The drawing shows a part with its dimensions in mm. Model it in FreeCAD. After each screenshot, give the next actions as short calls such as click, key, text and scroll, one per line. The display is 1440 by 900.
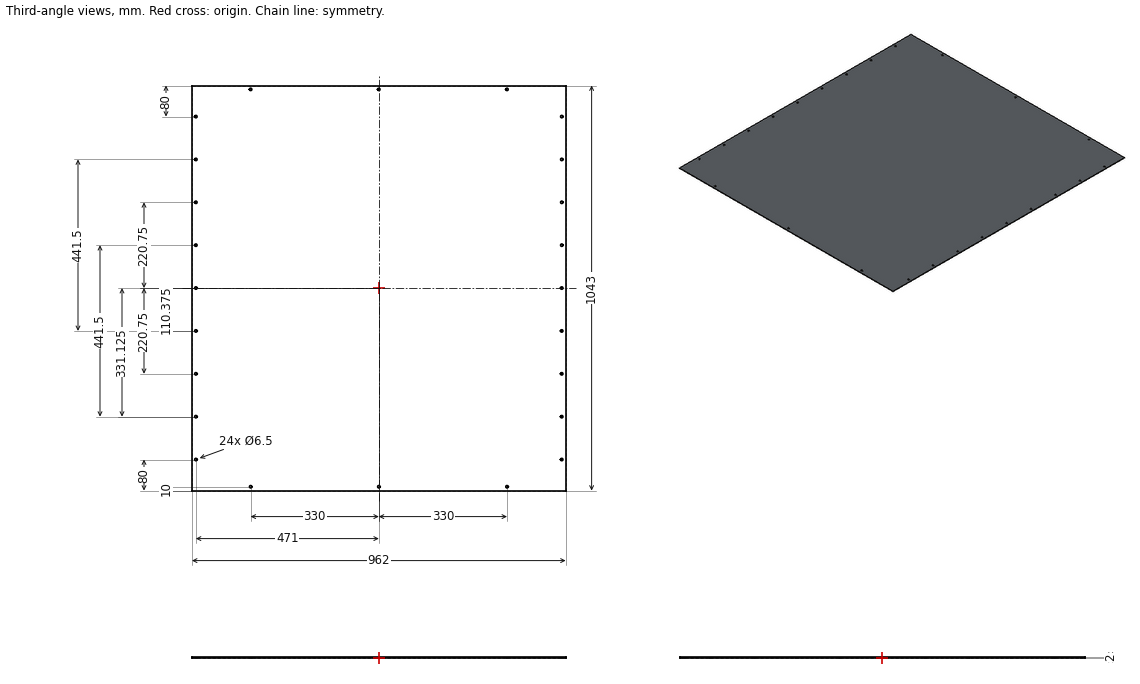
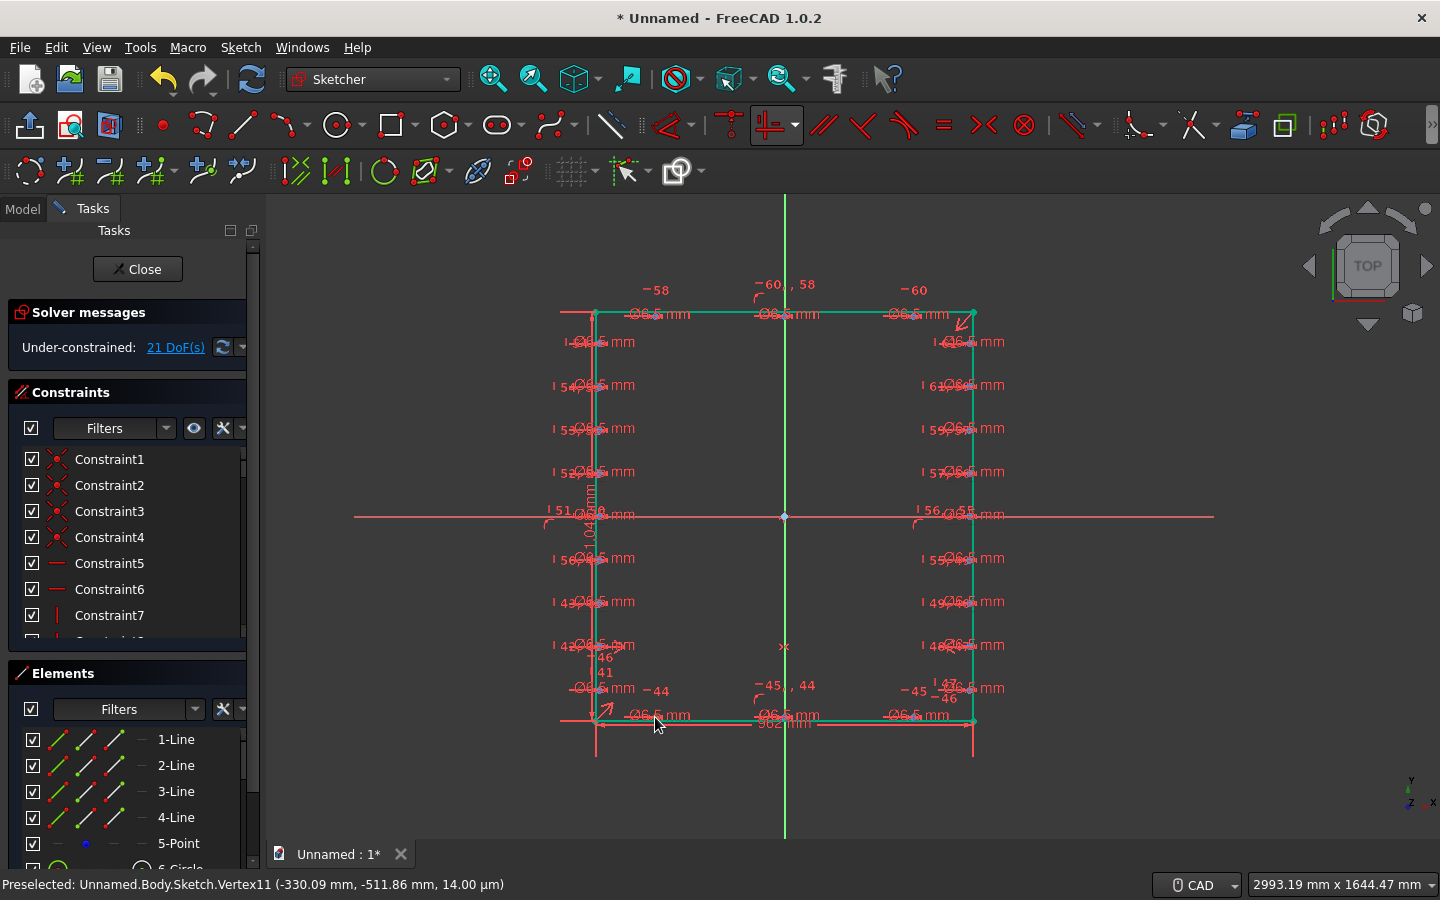
click(655, 316)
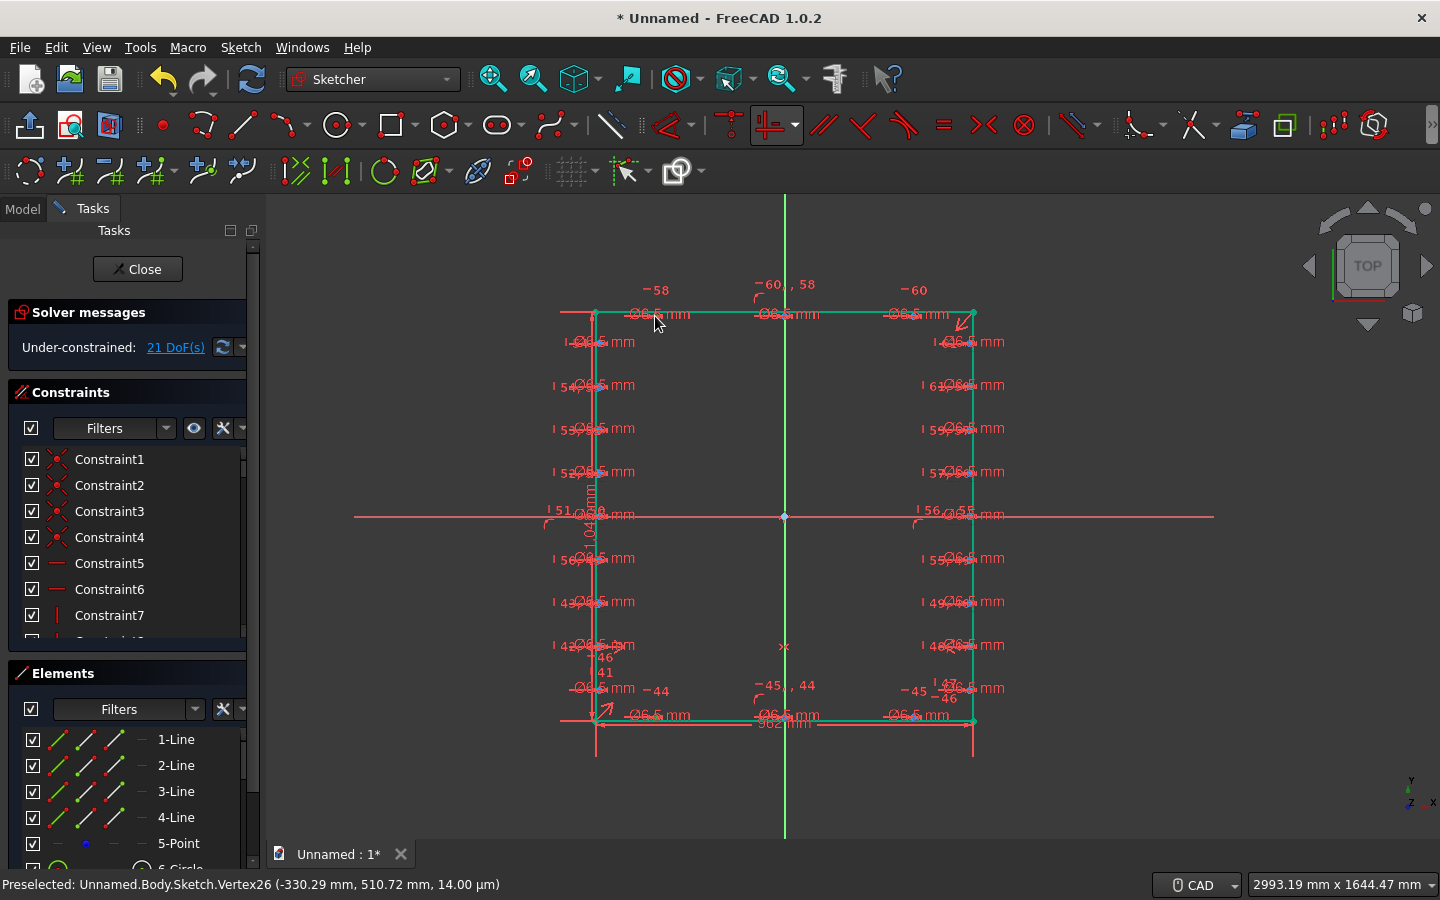
click(364, 517)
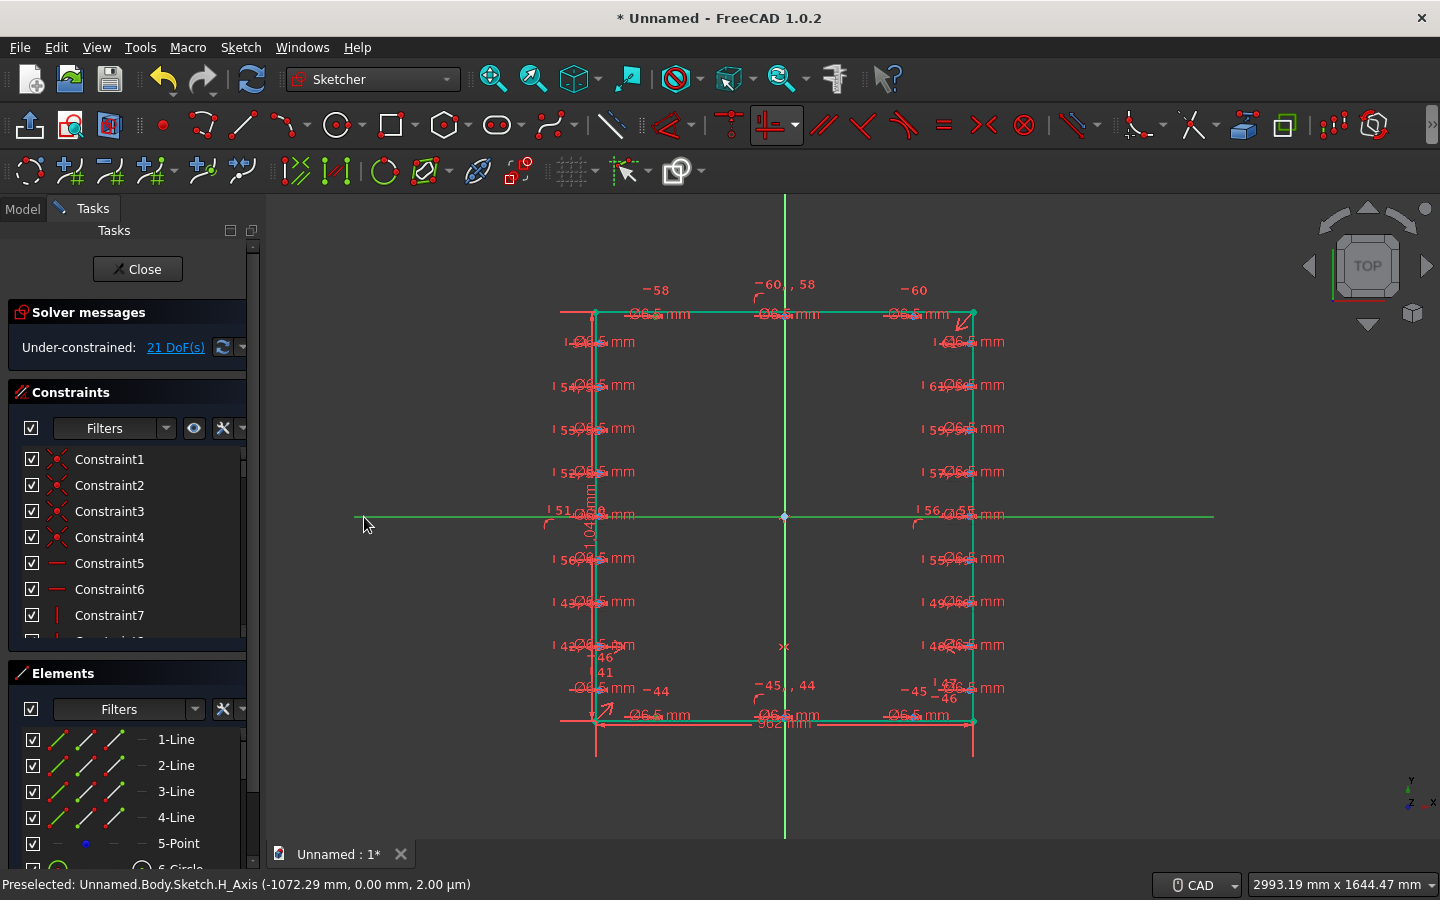
click(984, 126)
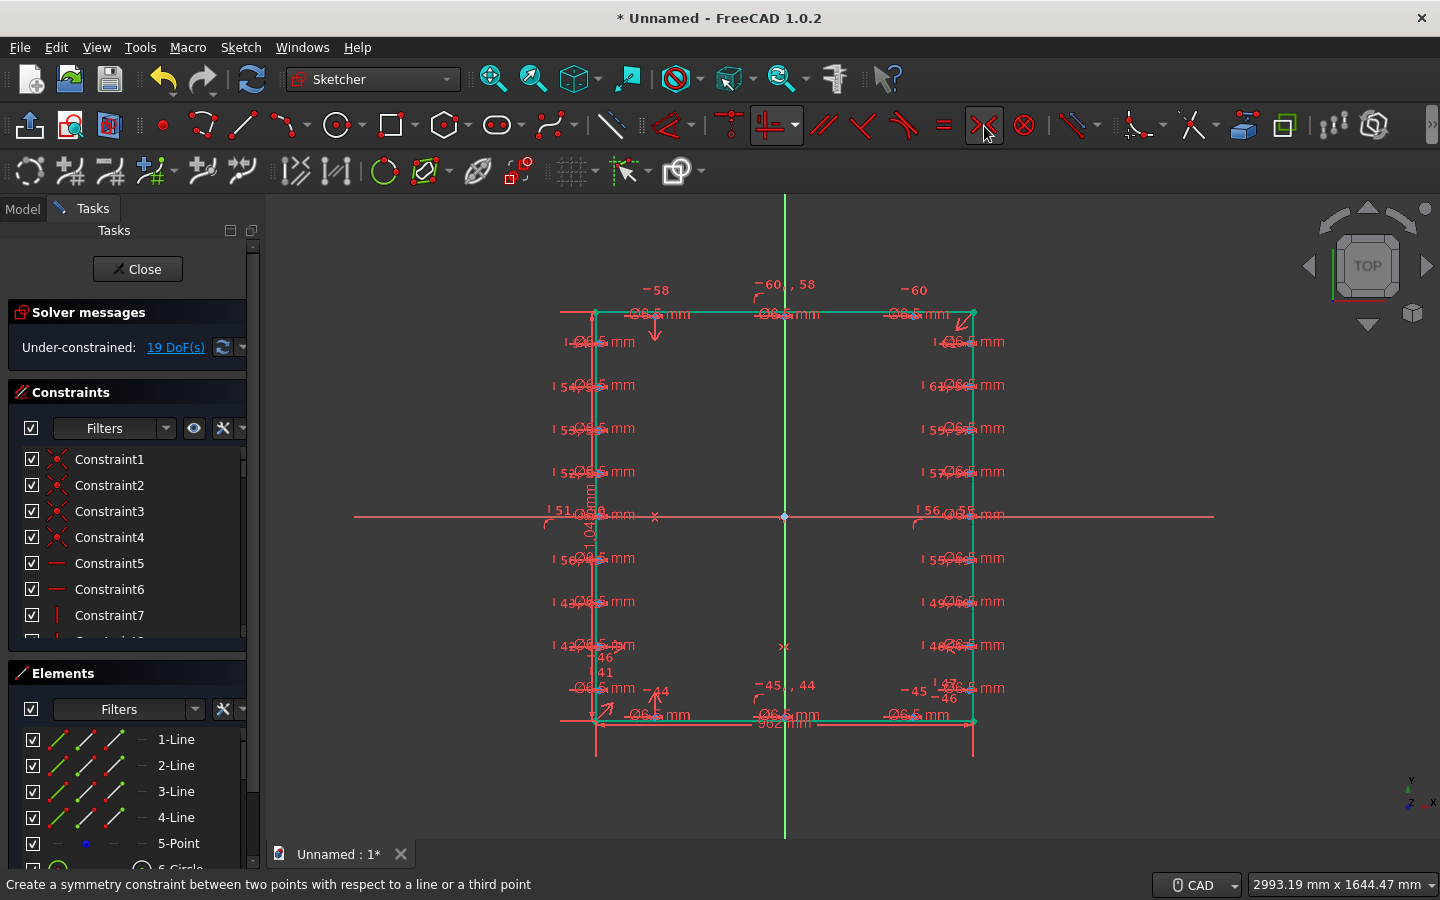
click(666, 126)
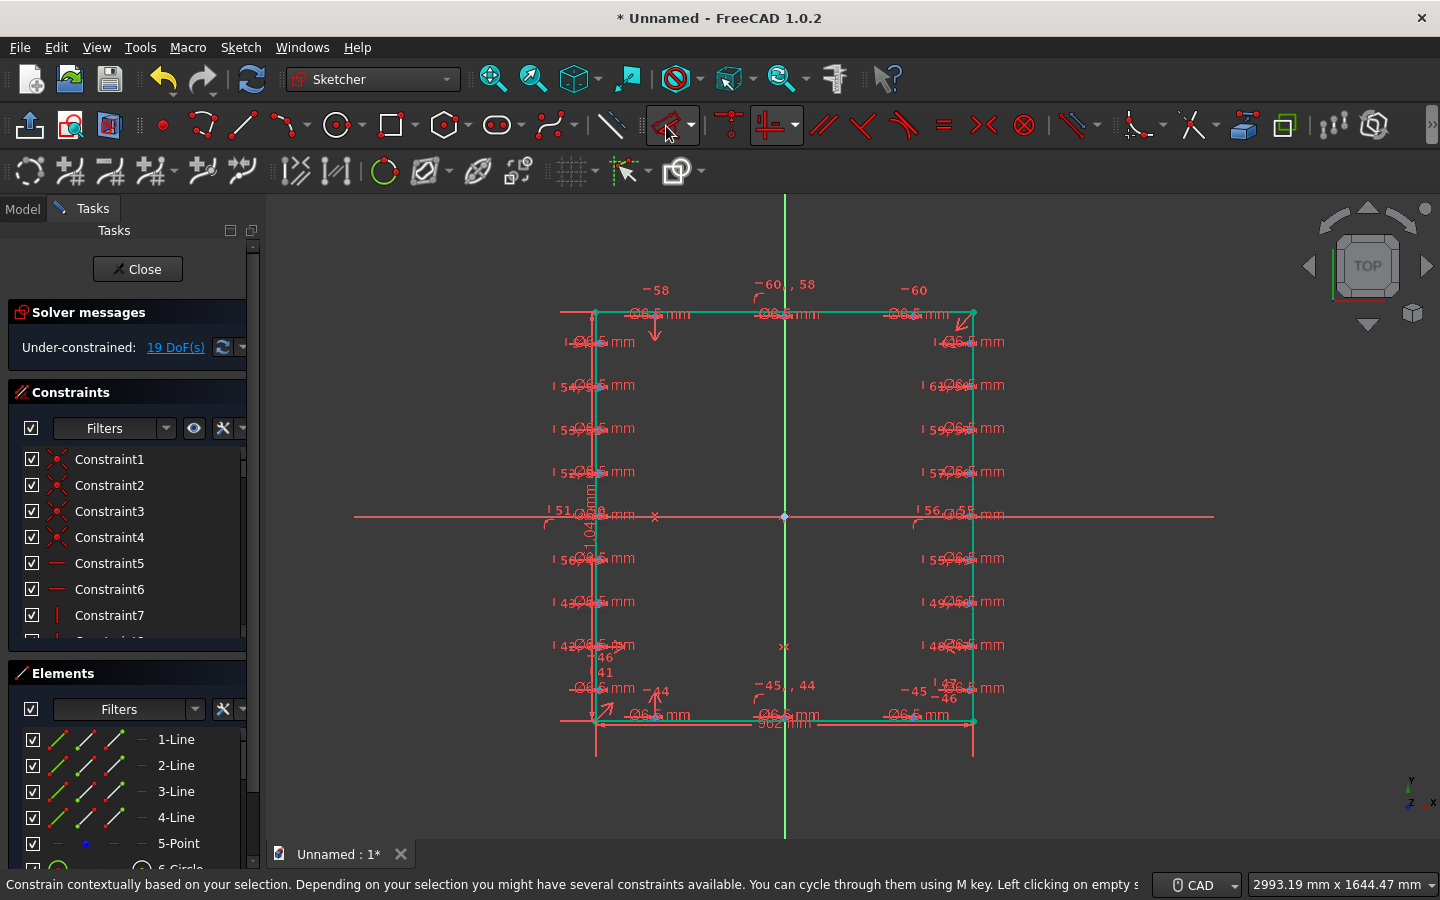
click(600, 690)
click(692, 483)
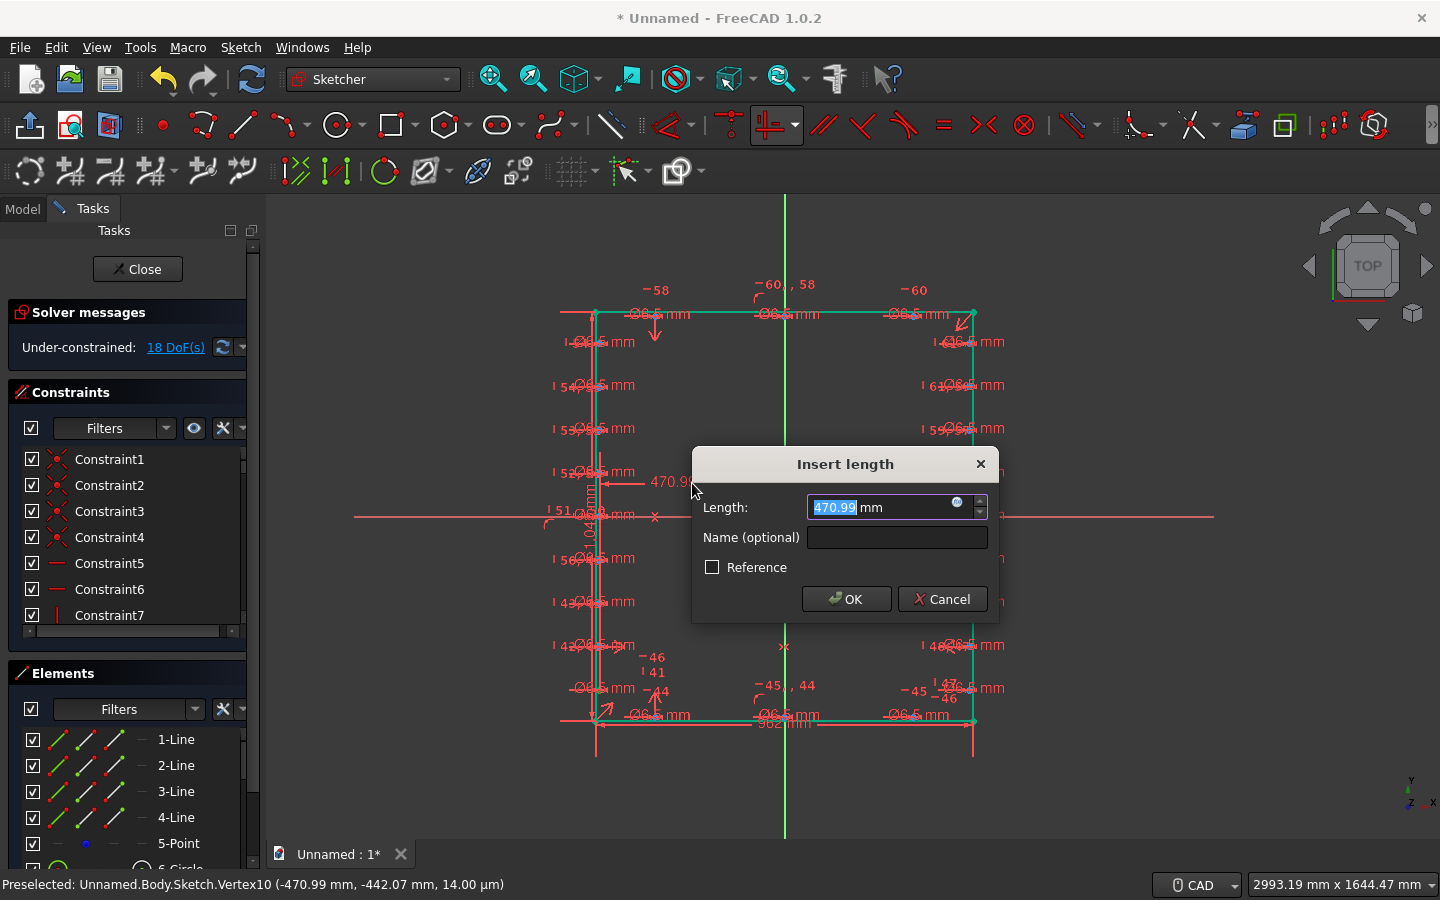
text(471)
key(Return)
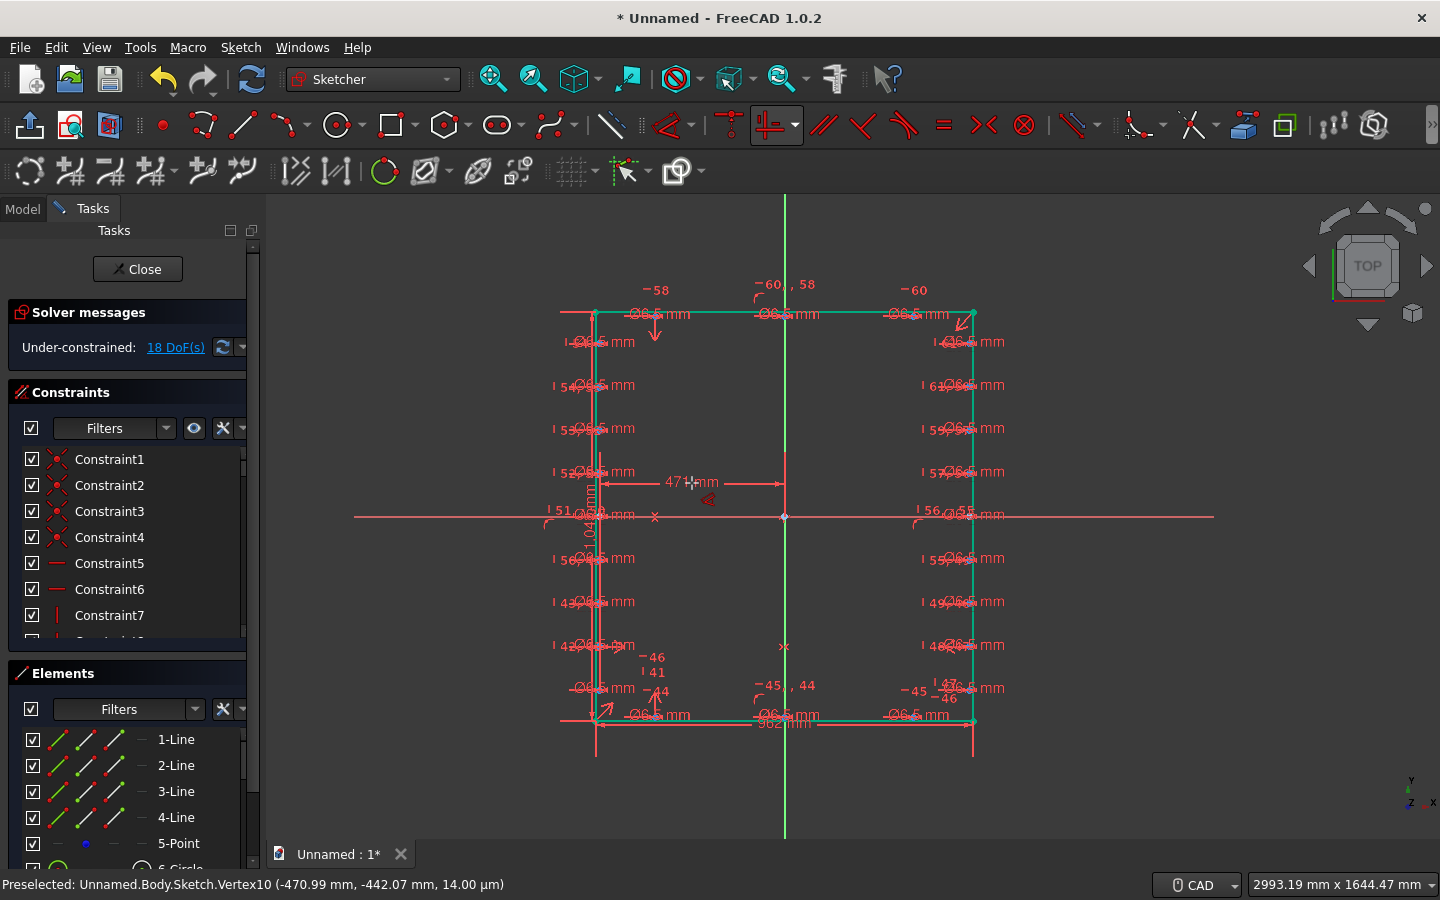
click(655, 717)
click(720, 751)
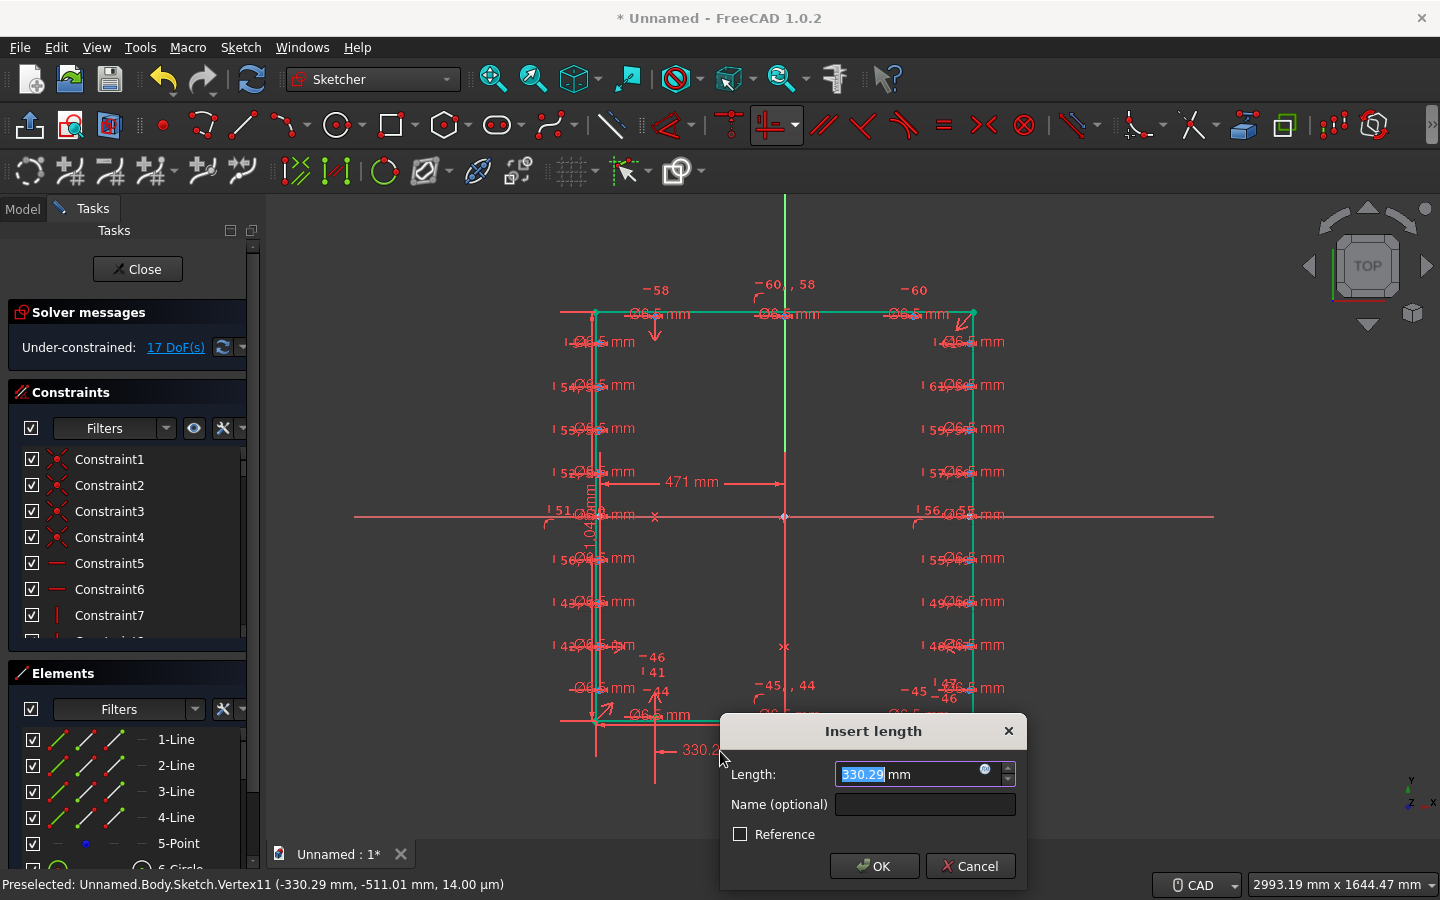
text(330)
key(Return)